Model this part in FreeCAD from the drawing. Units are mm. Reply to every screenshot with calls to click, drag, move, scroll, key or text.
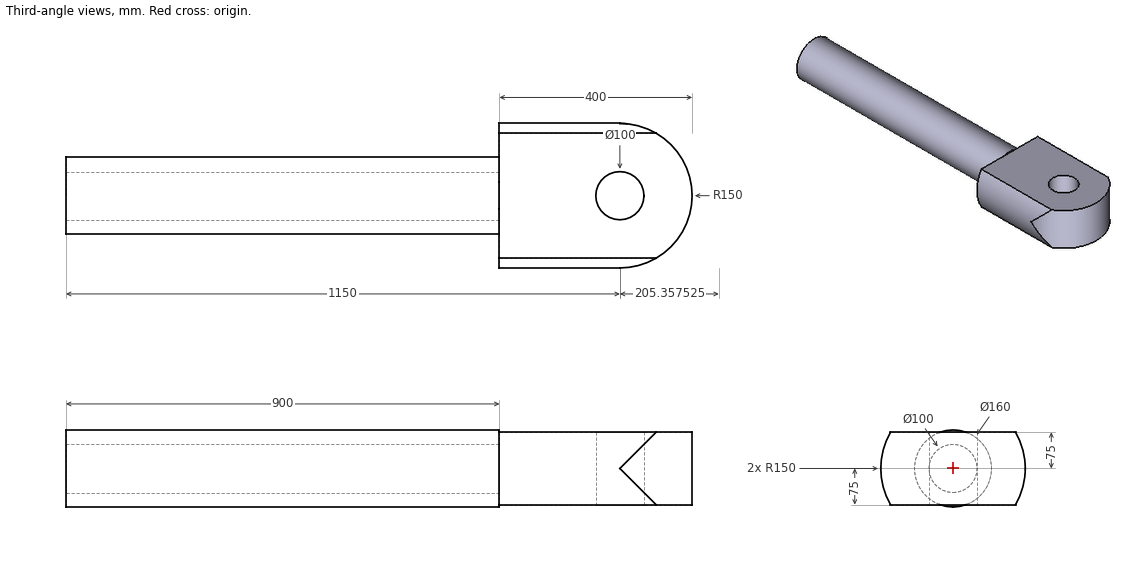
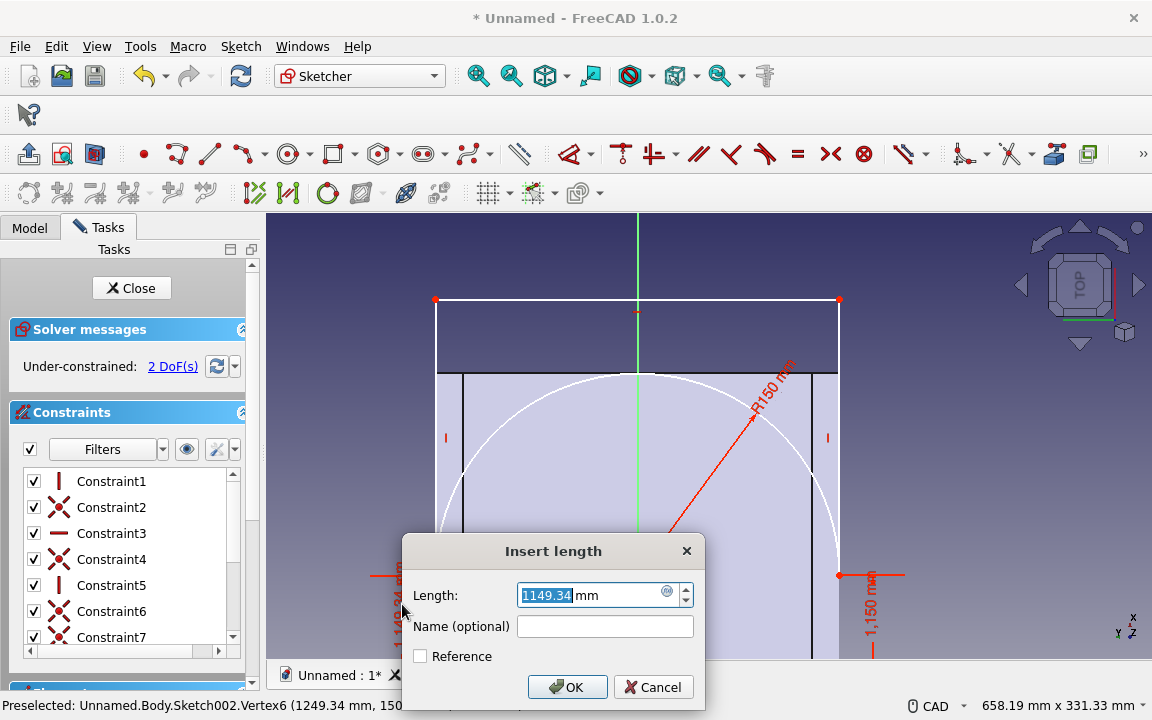
text(1150)
key(Return)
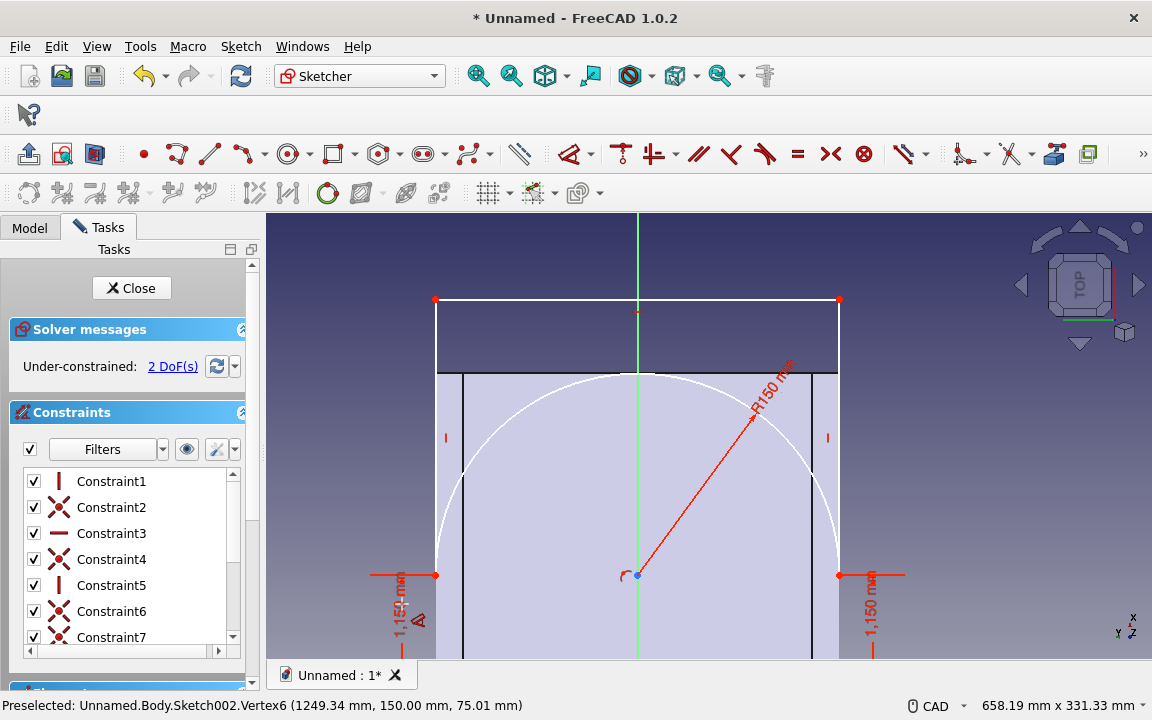
click(638, 576)
click(672, 603)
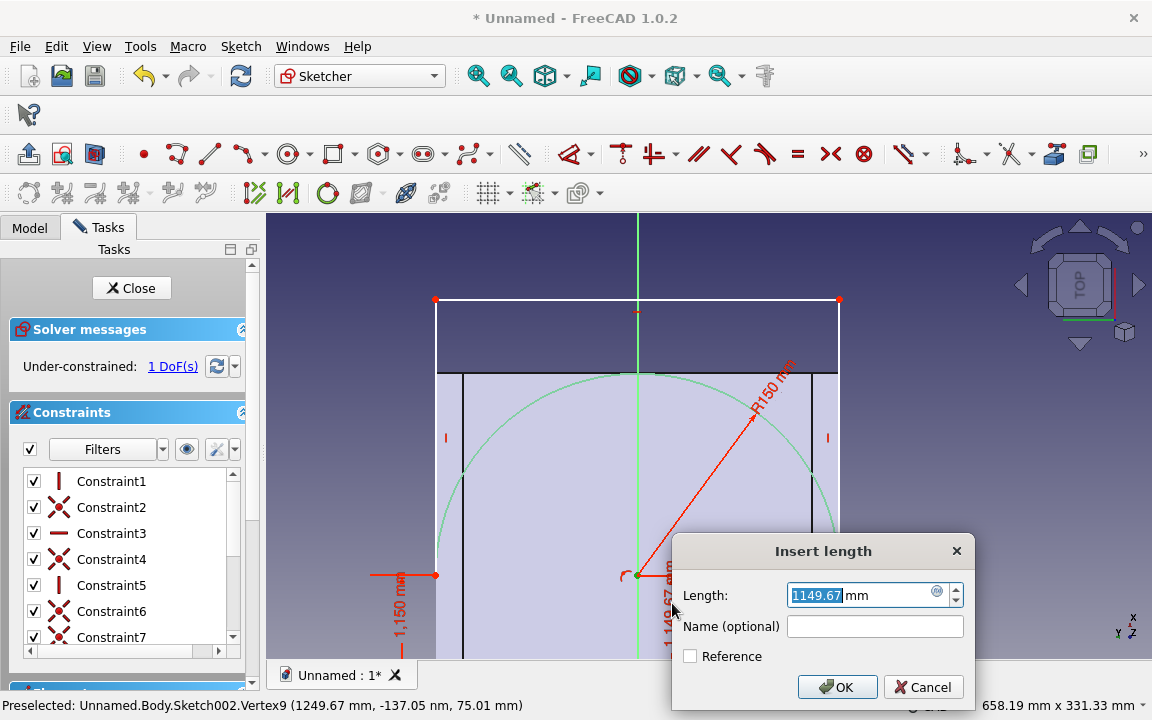
text(1150)
key(Return)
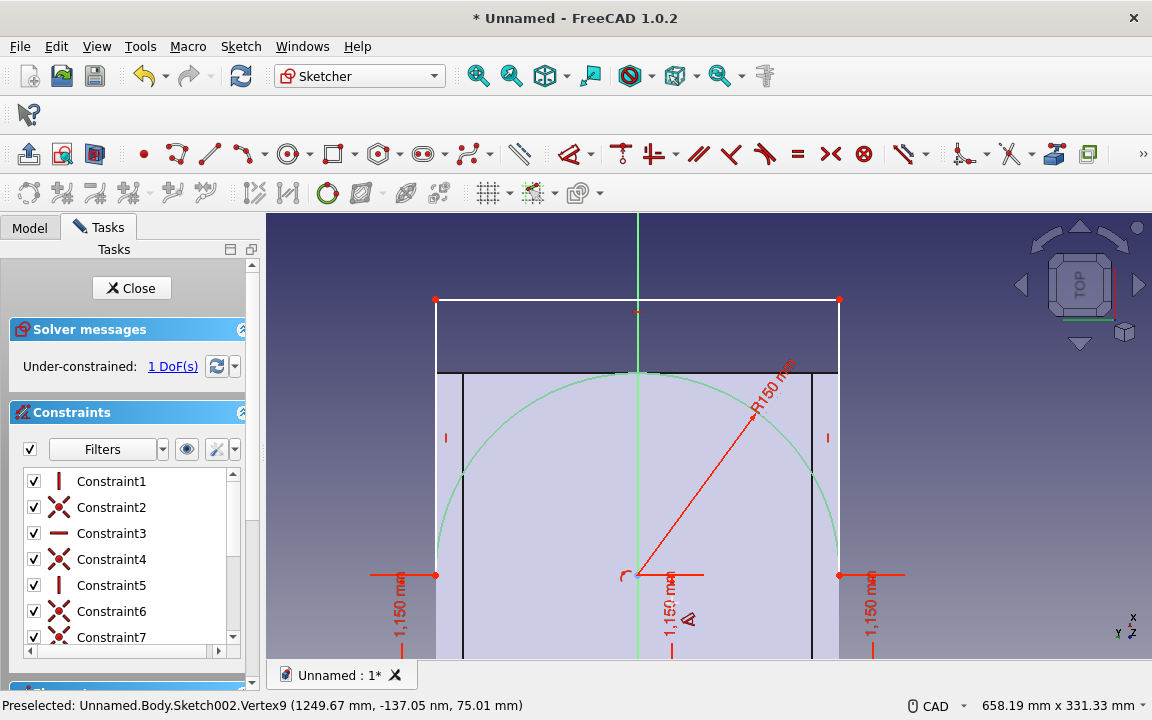
click(839, 493)
click(873, 438)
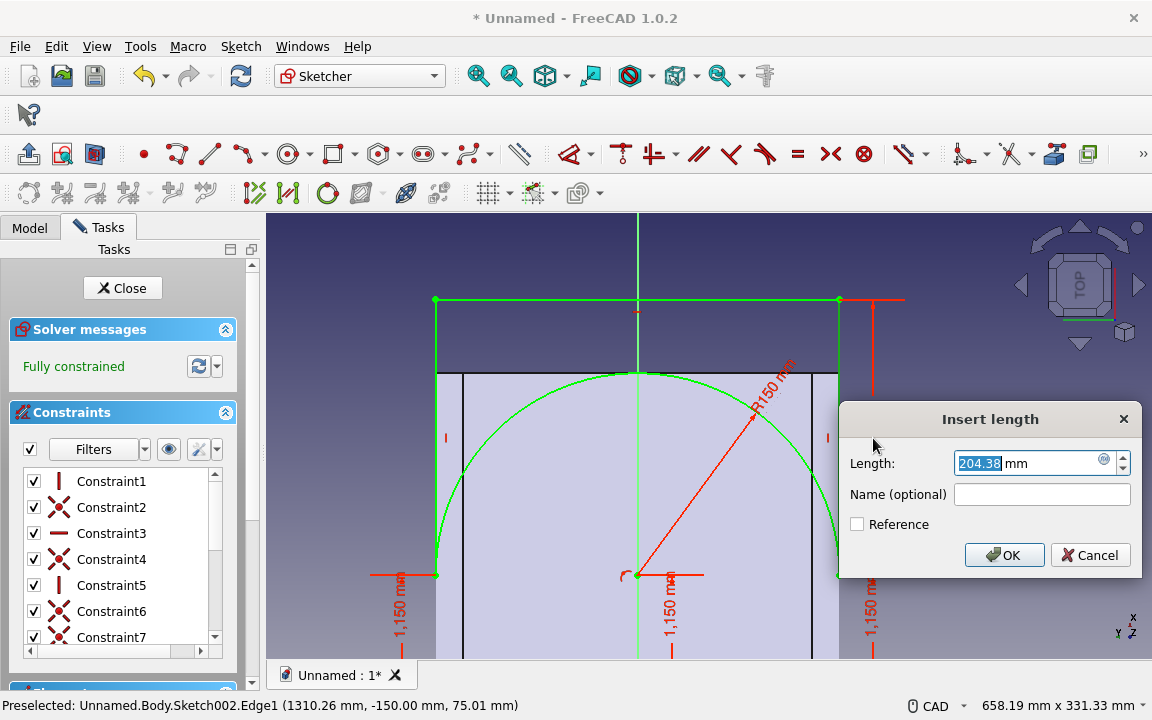
text(205.357525)
key(Return)
key(Escape)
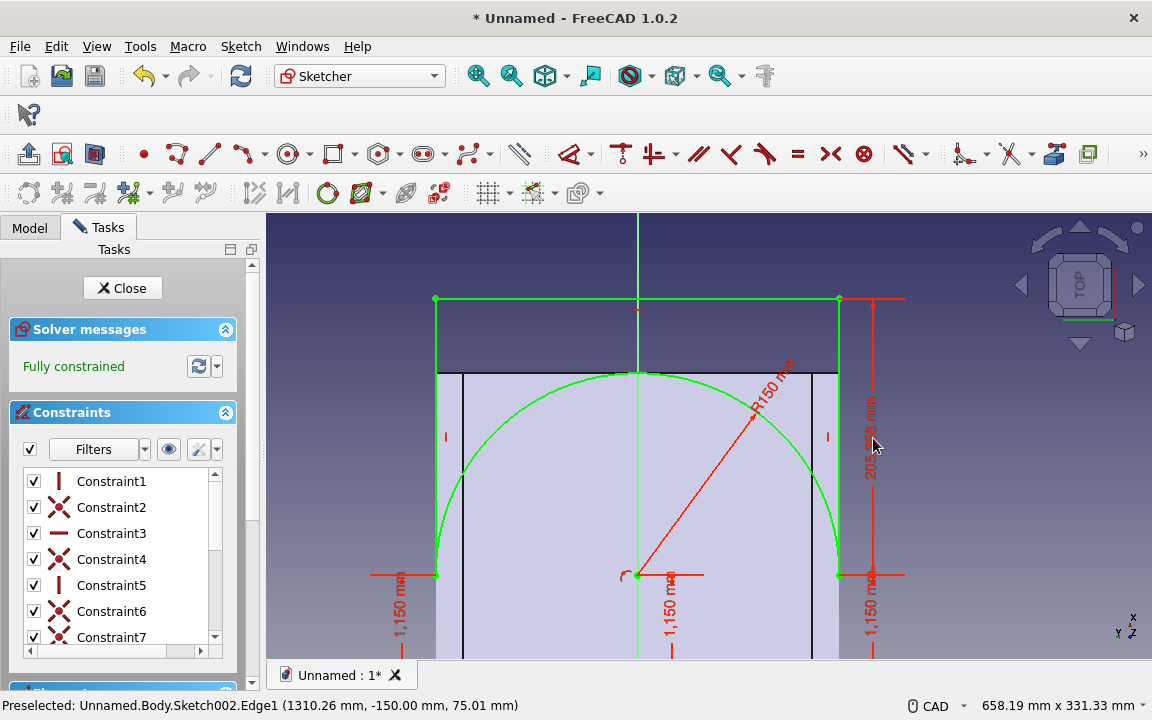
click(123, 288)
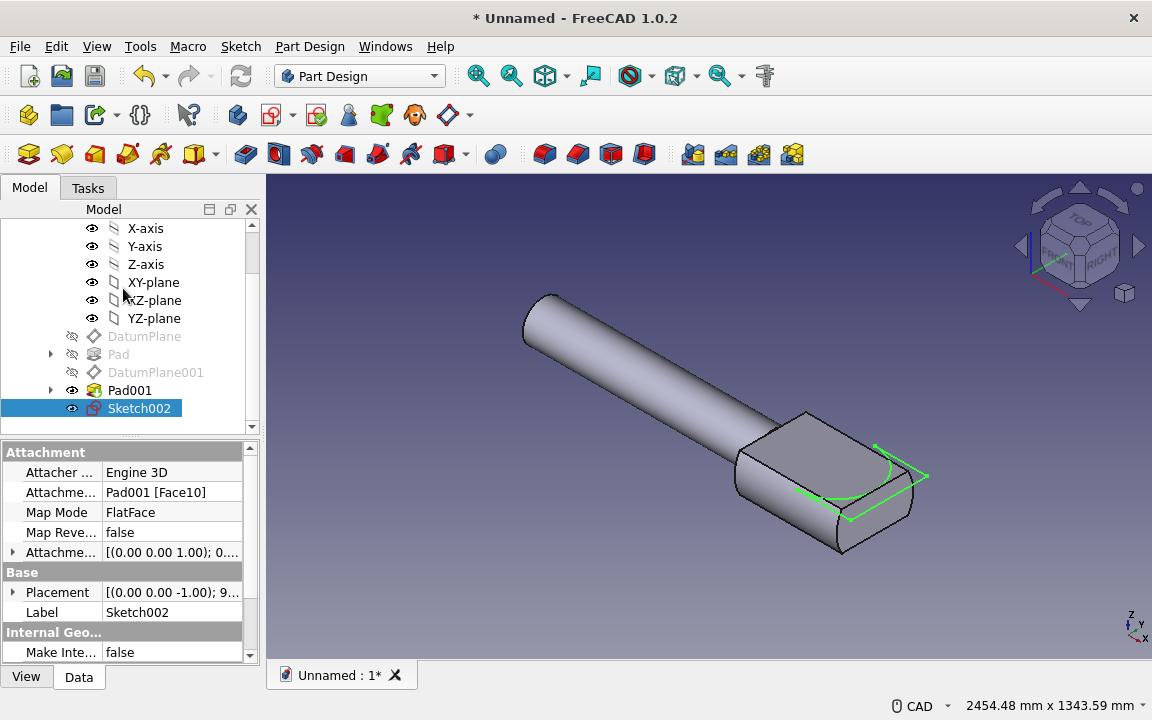
click(246, 154)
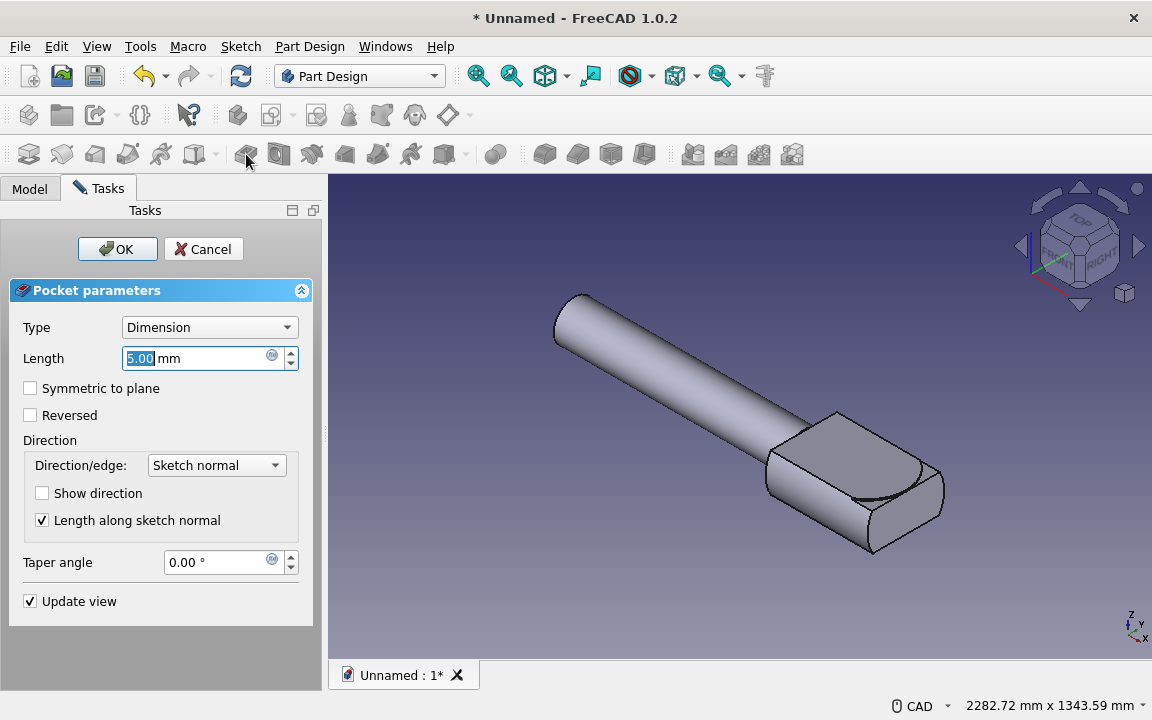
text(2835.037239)
key(Tab)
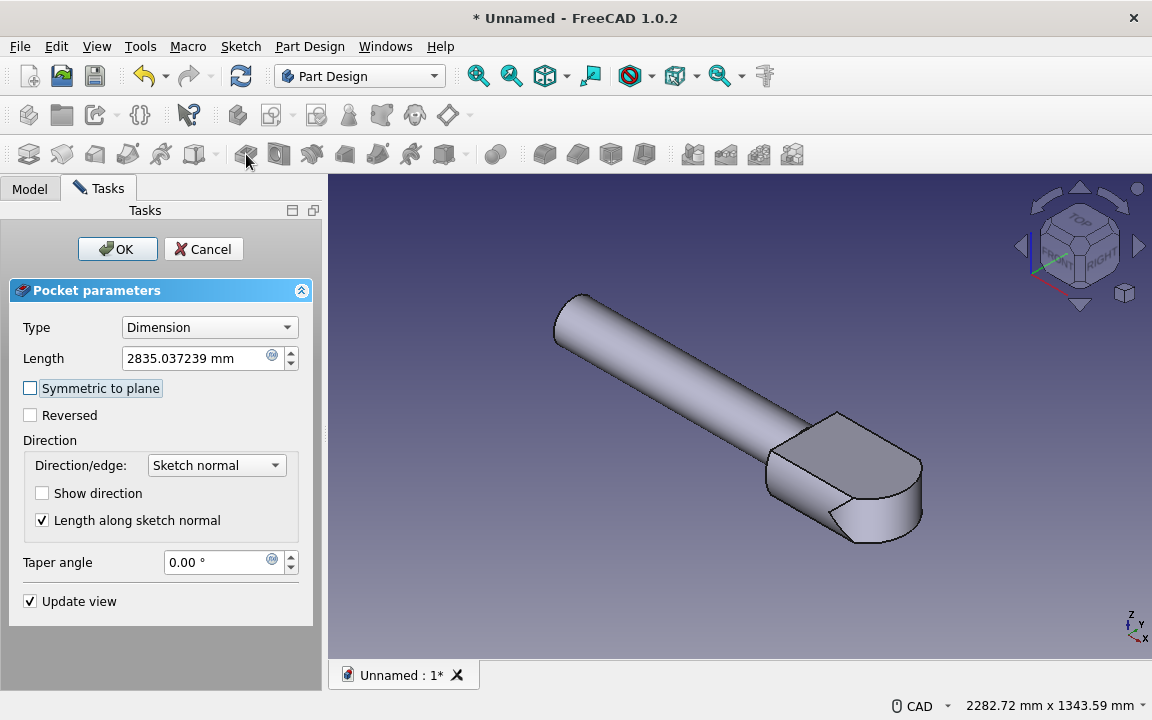
click(31, 388)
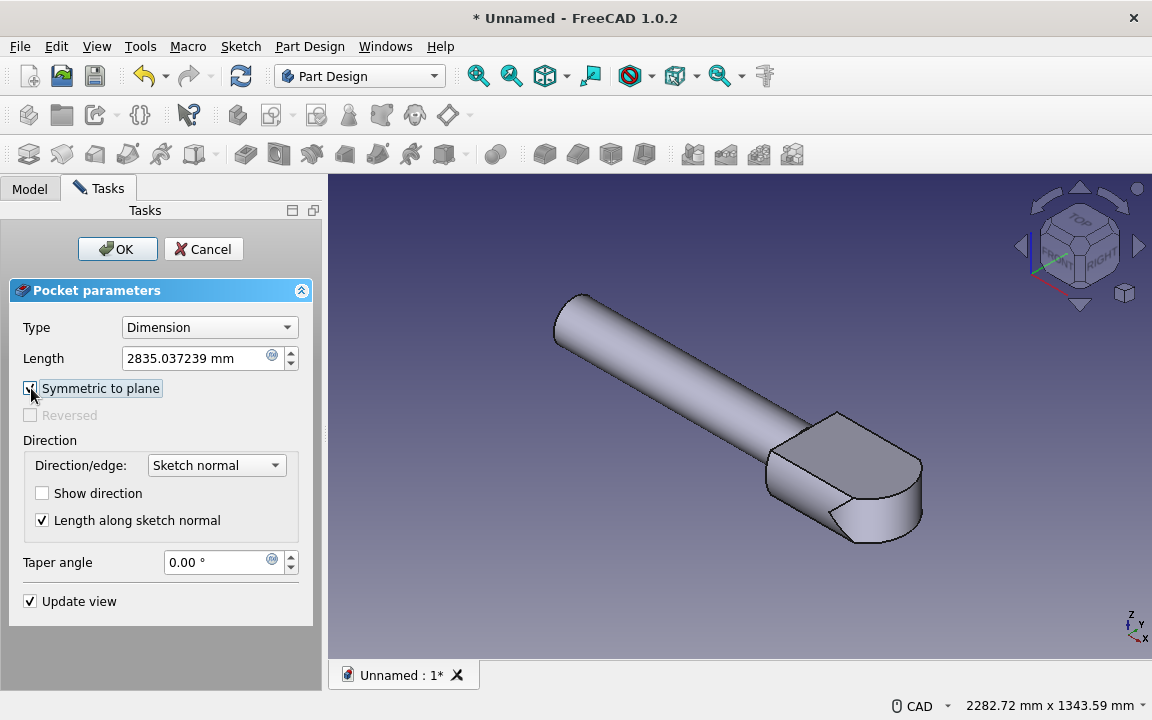
click(118, 249)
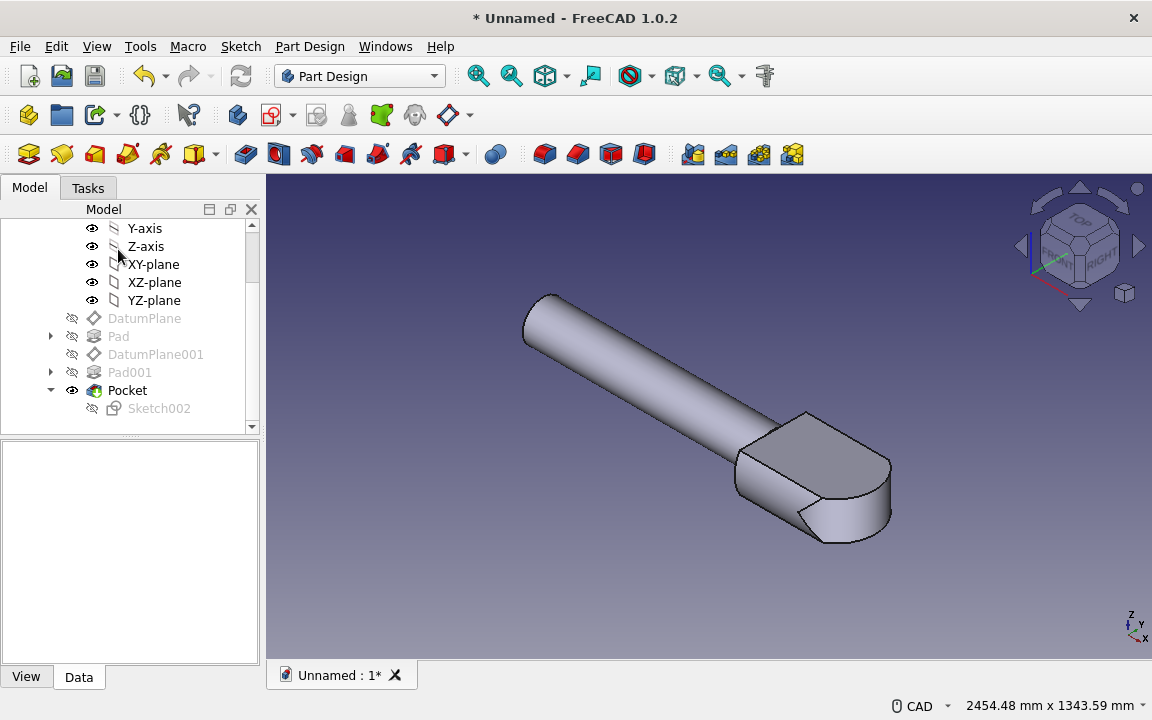
click(838, 468)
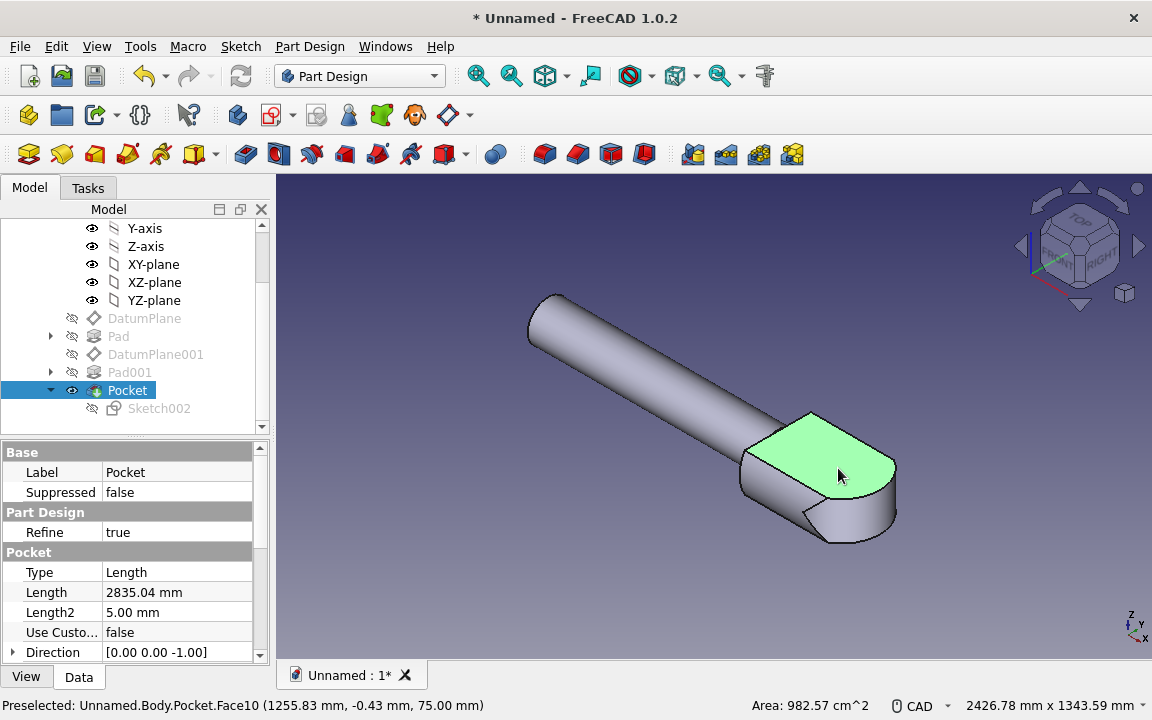
click(270, 116)